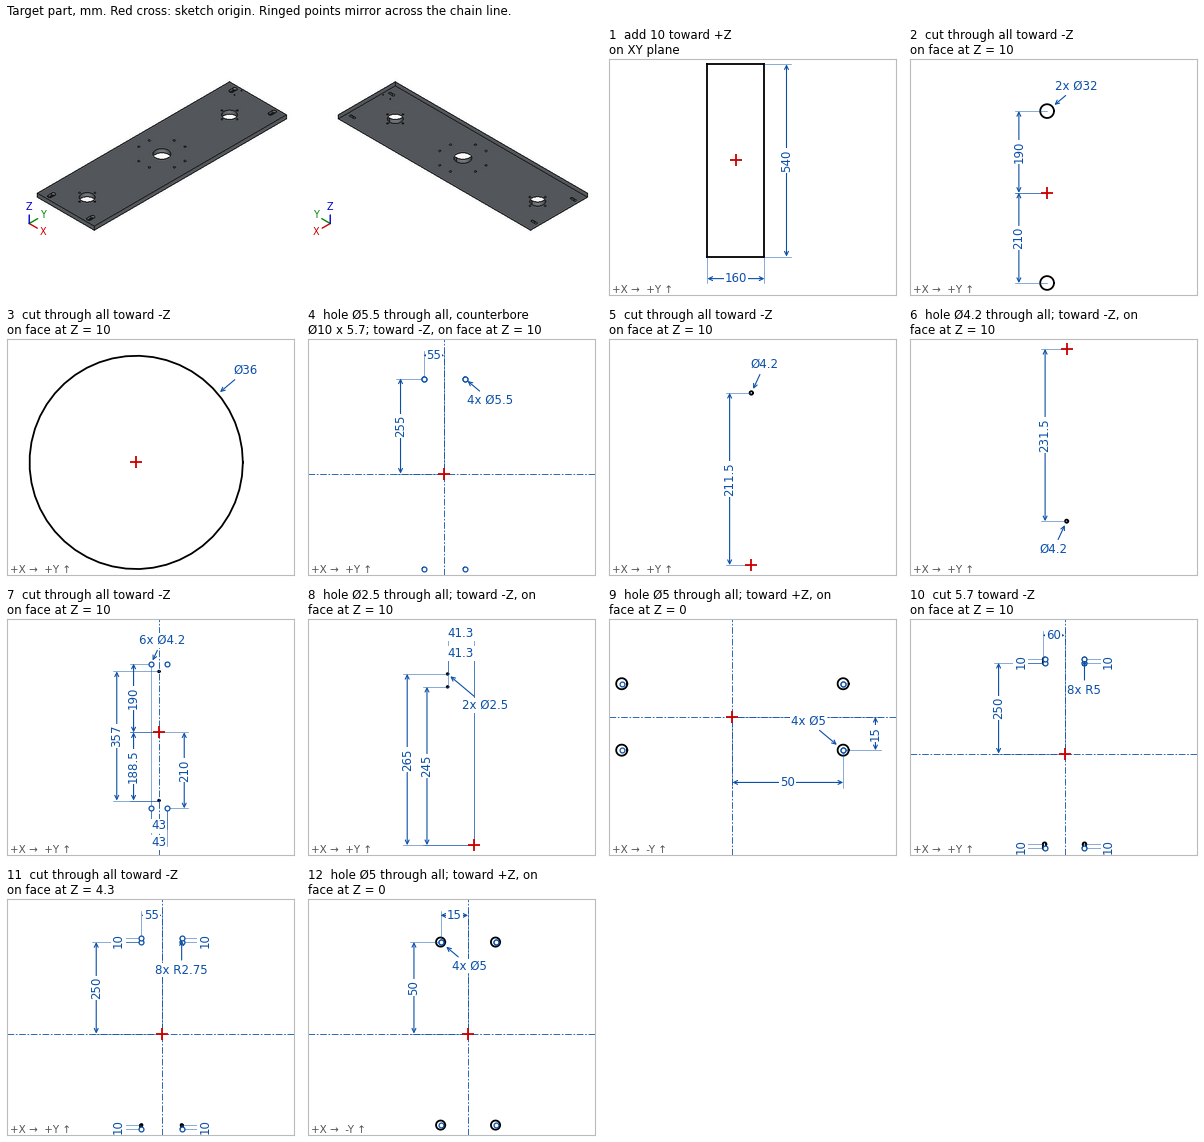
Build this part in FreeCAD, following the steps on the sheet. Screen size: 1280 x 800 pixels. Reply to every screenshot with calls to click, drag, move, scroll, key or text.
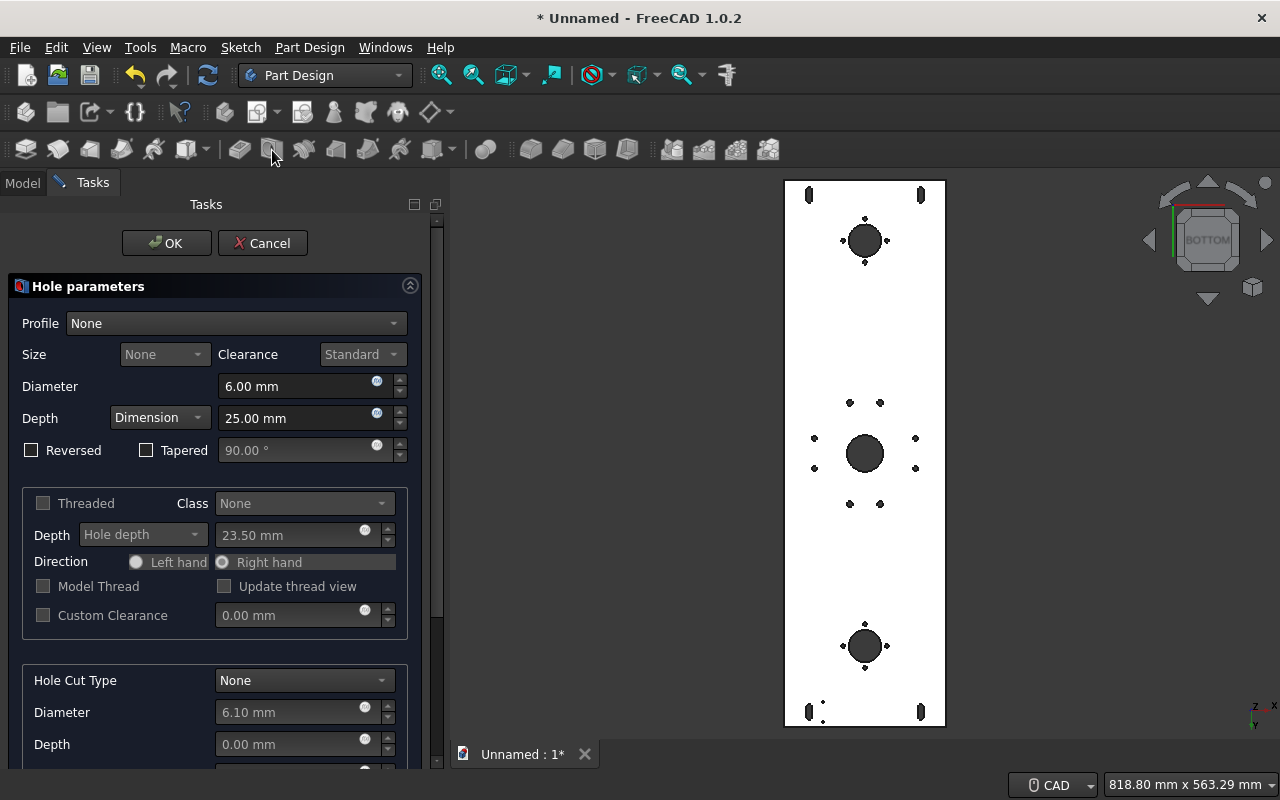
triple_click(305, 386)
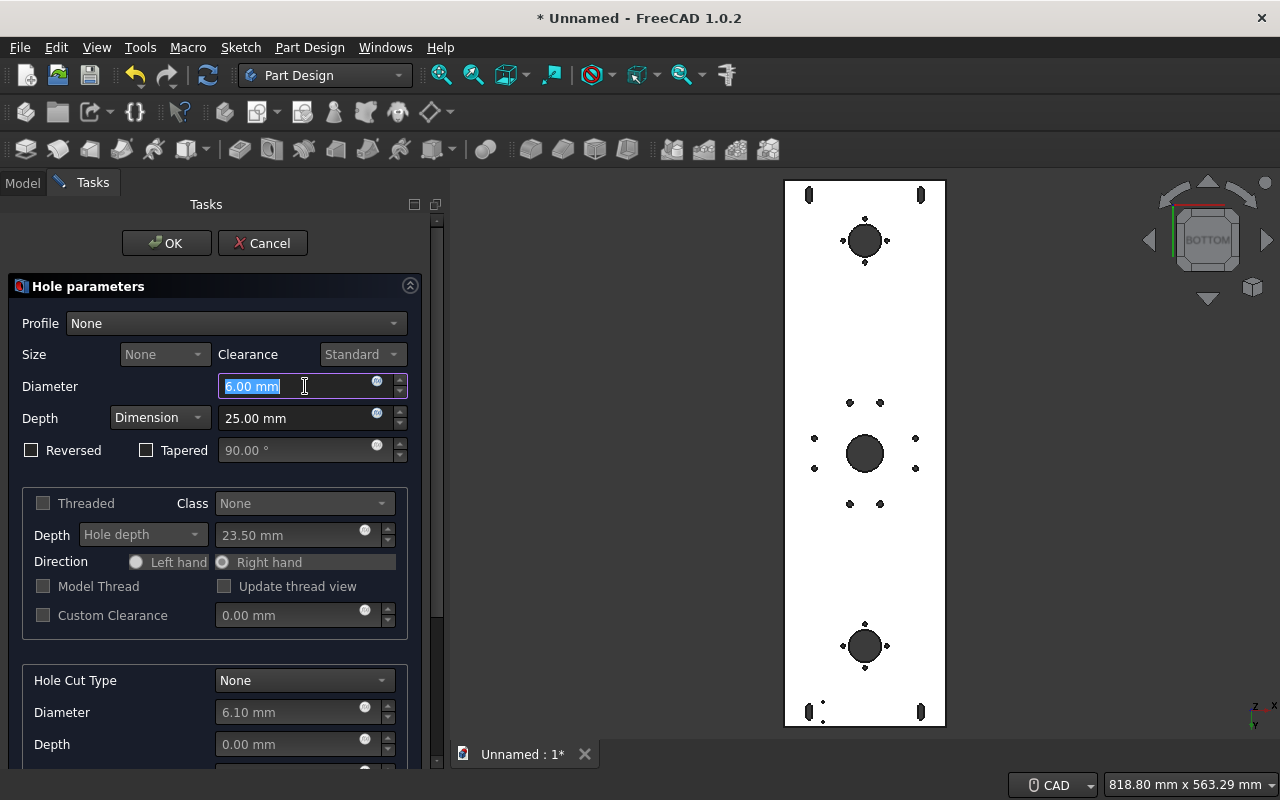
text(5)
key(Tab)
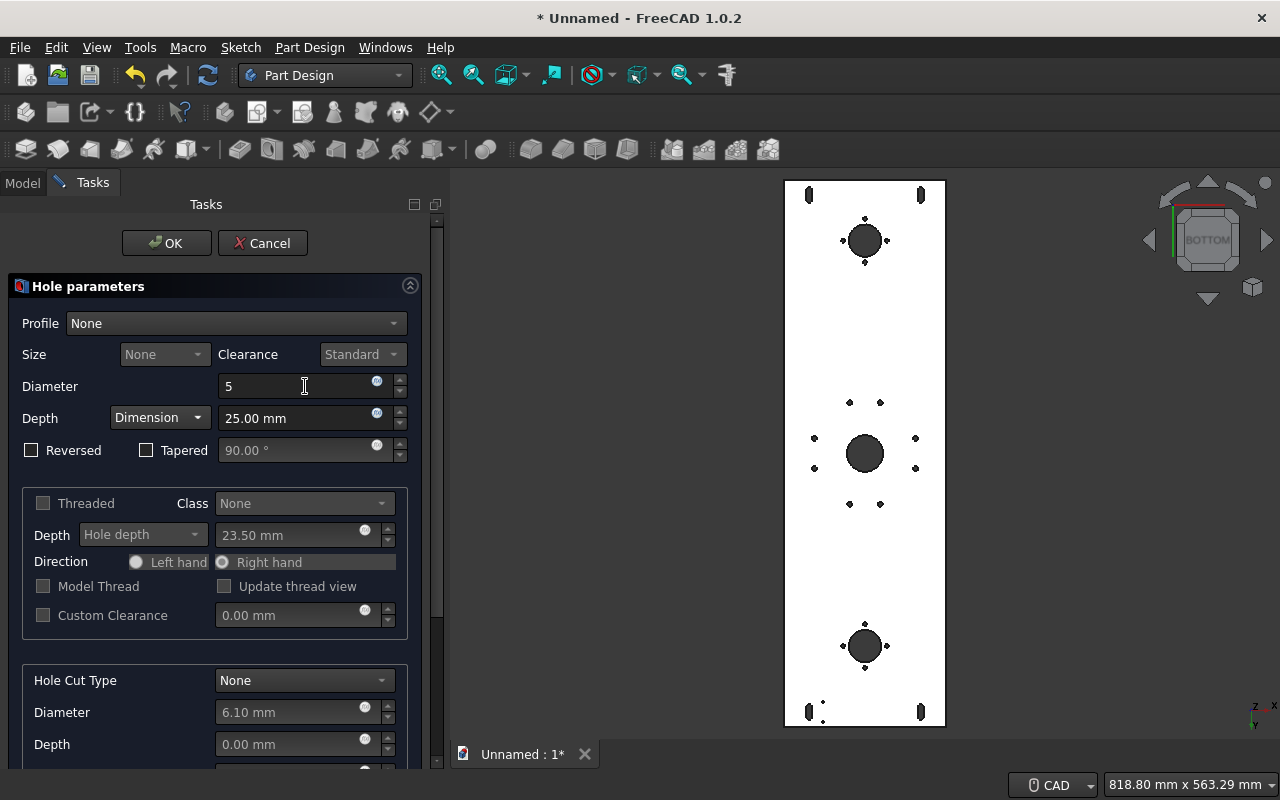
click(161, 418)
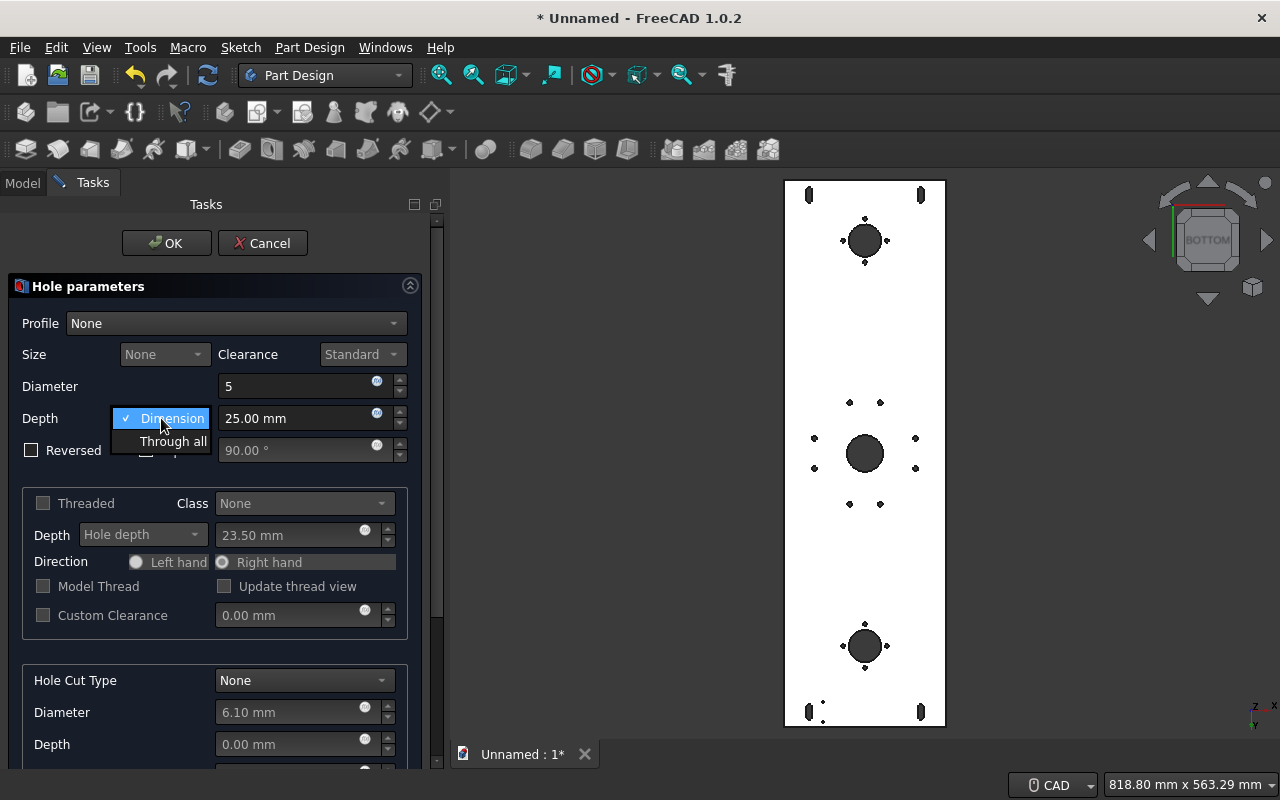
click(160, 442)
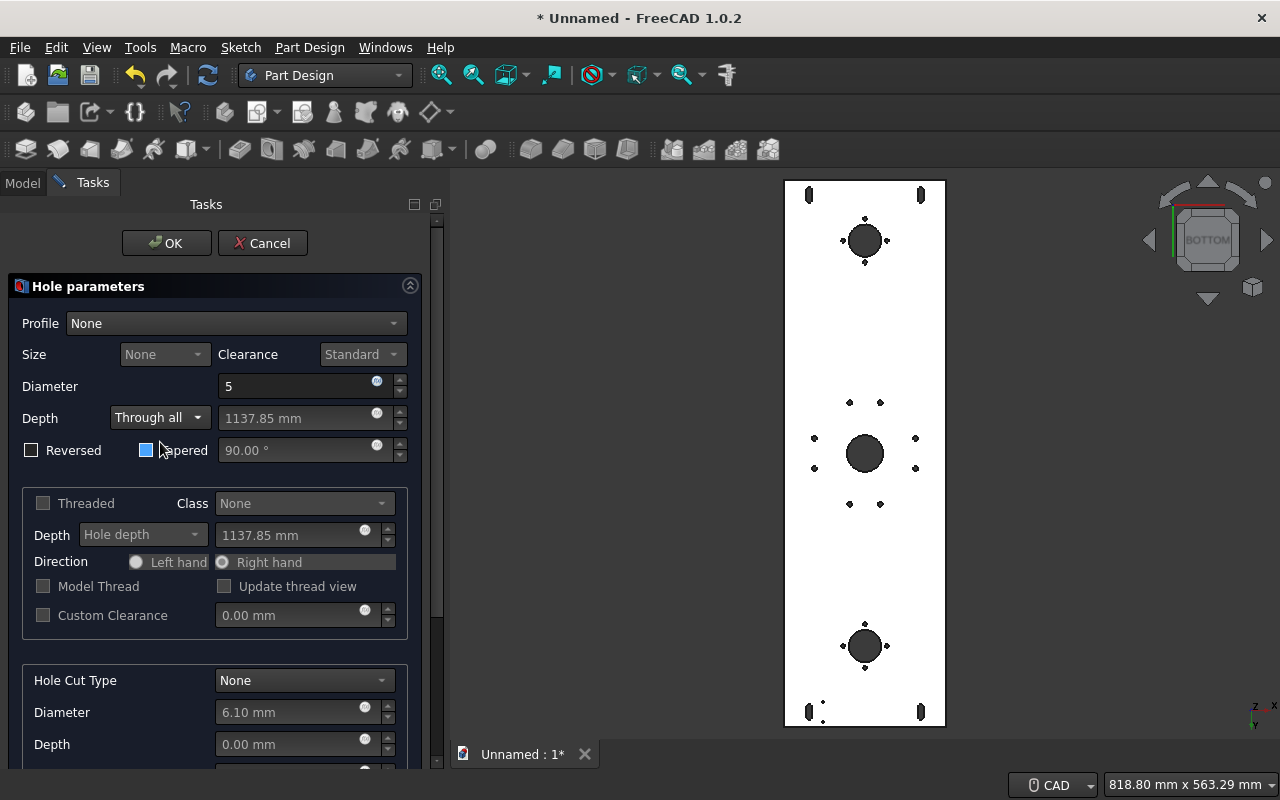
click(167, 243)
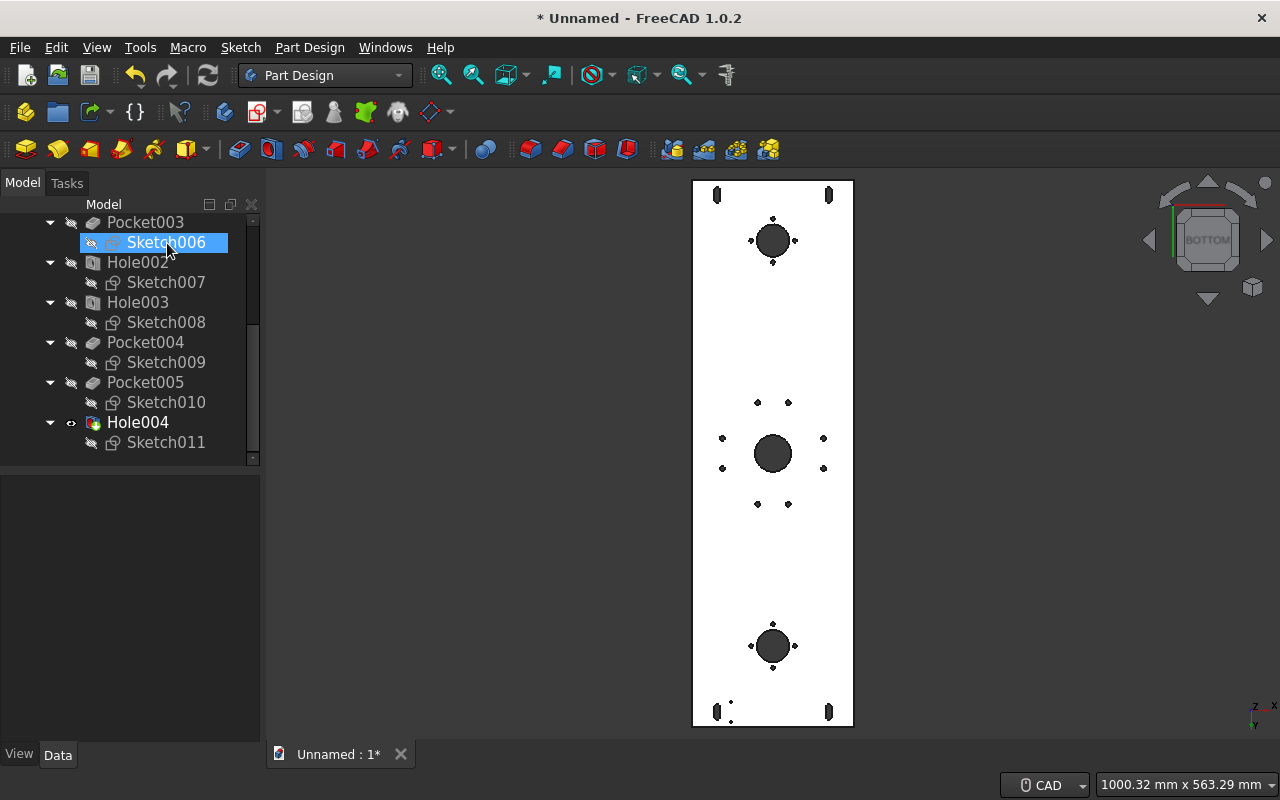
key(0)